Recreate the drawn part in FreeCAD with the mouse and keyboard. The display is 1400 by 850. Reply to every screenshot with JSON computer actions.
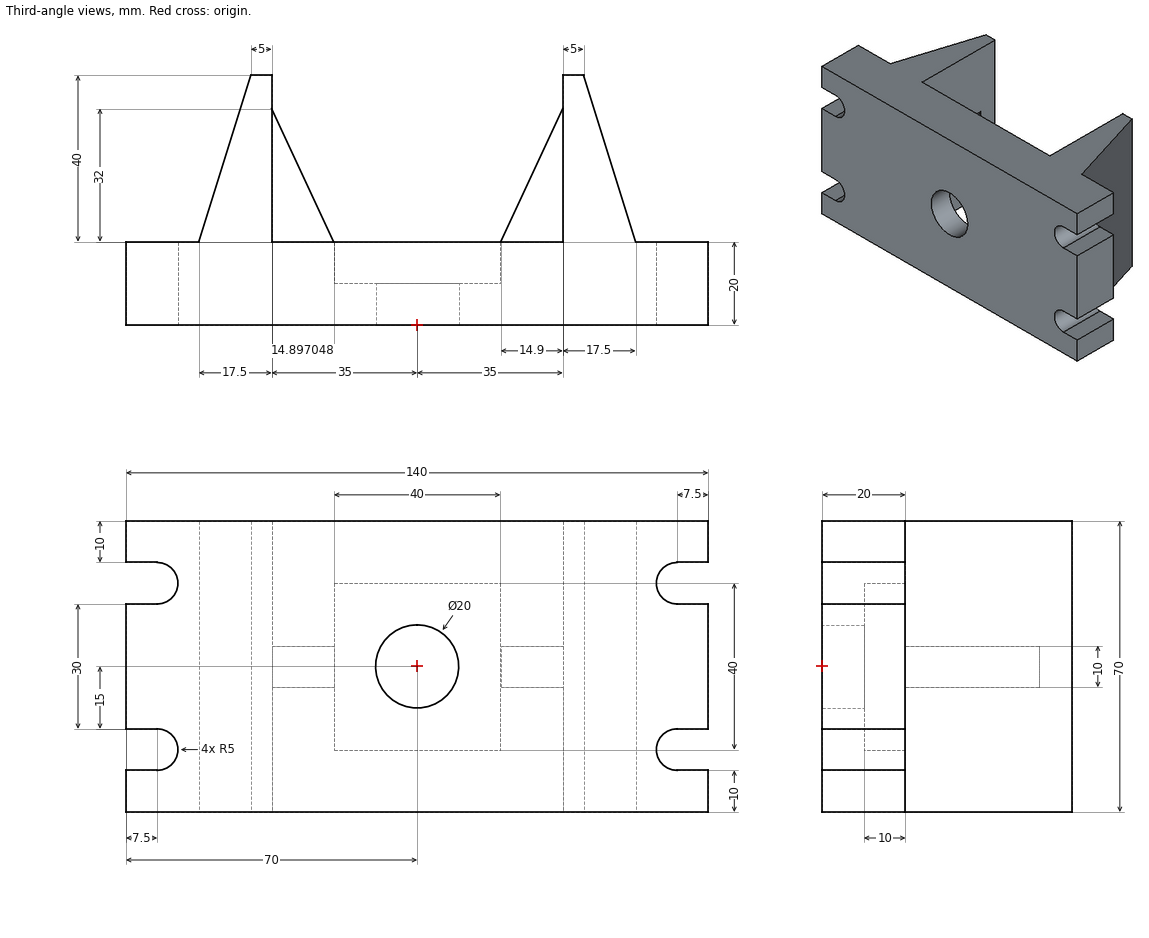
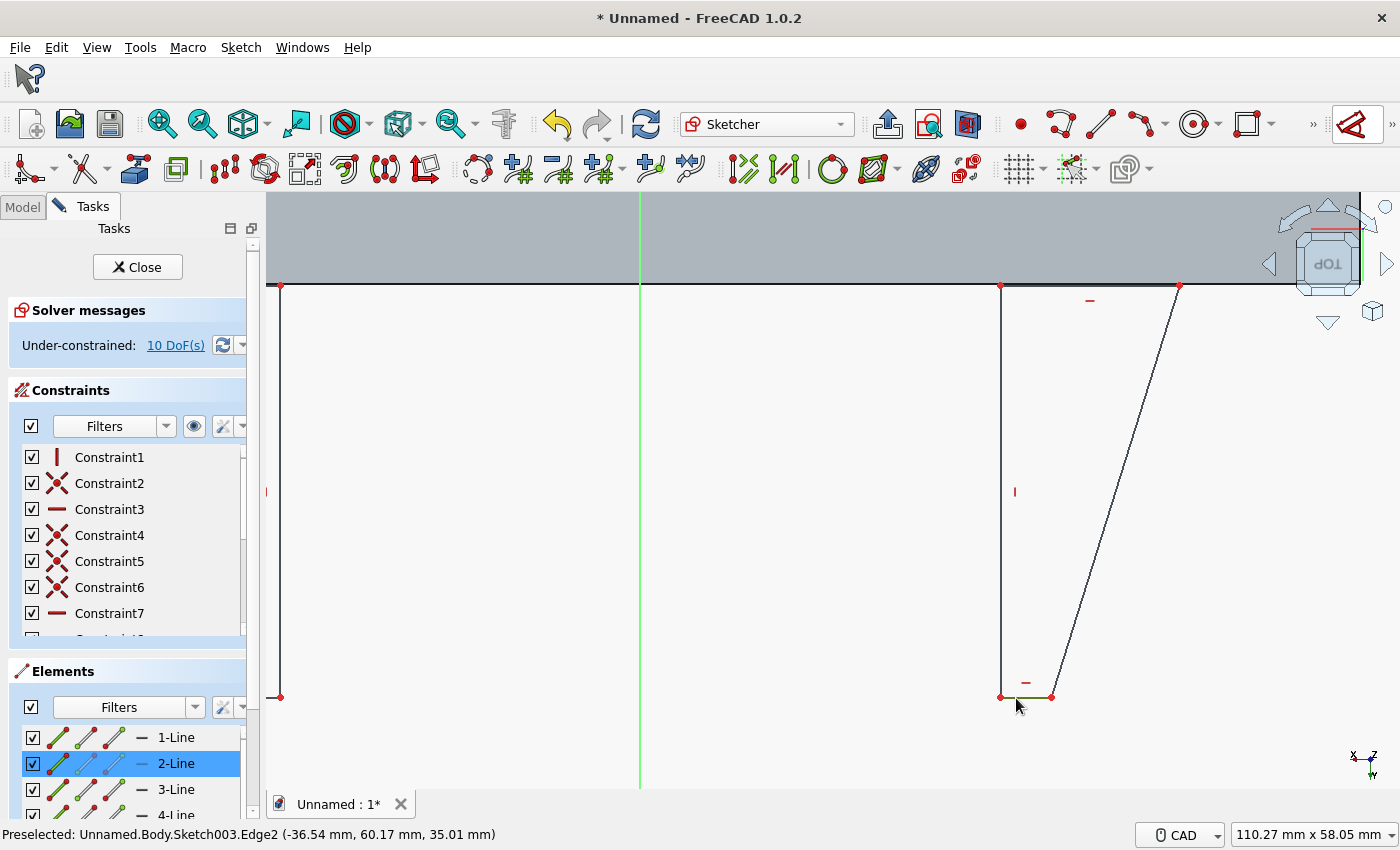
{"action": "left_click", "coordinate": [1378, 124]}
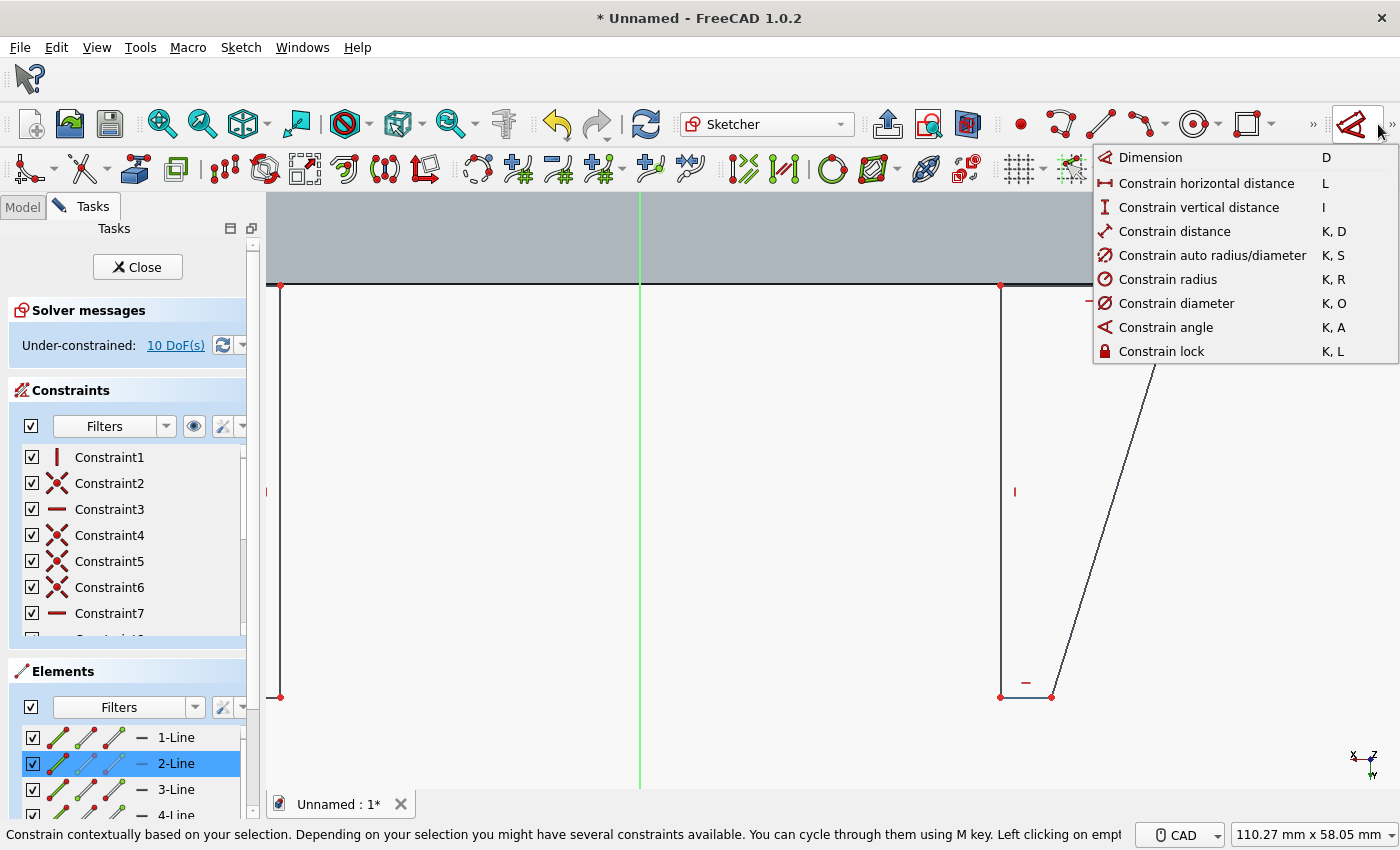
{"action": "left_click", "coordinate": [1246, 183]}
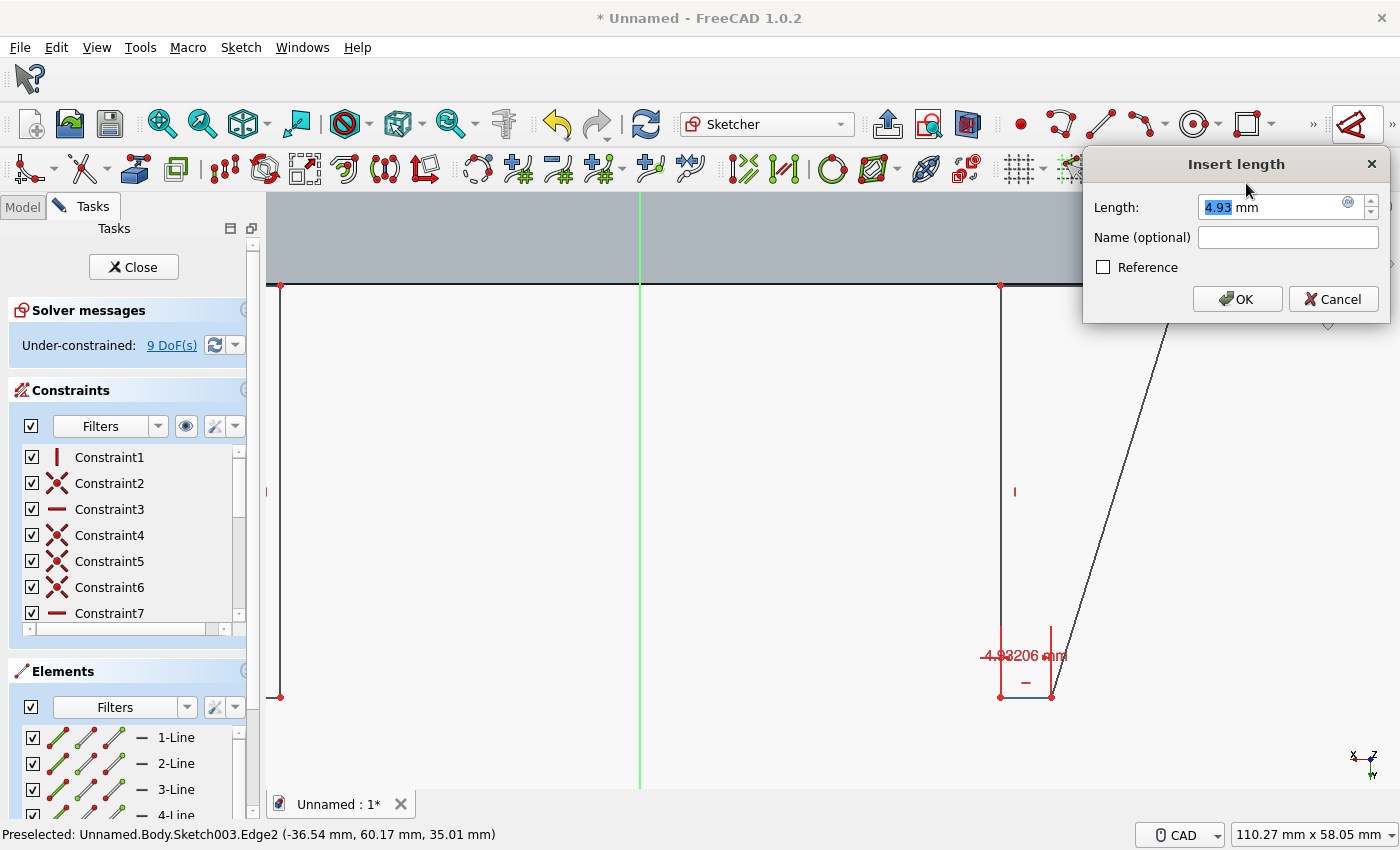
{"action": "type", "text": "5"}
{"action": "key", "text": "Return"}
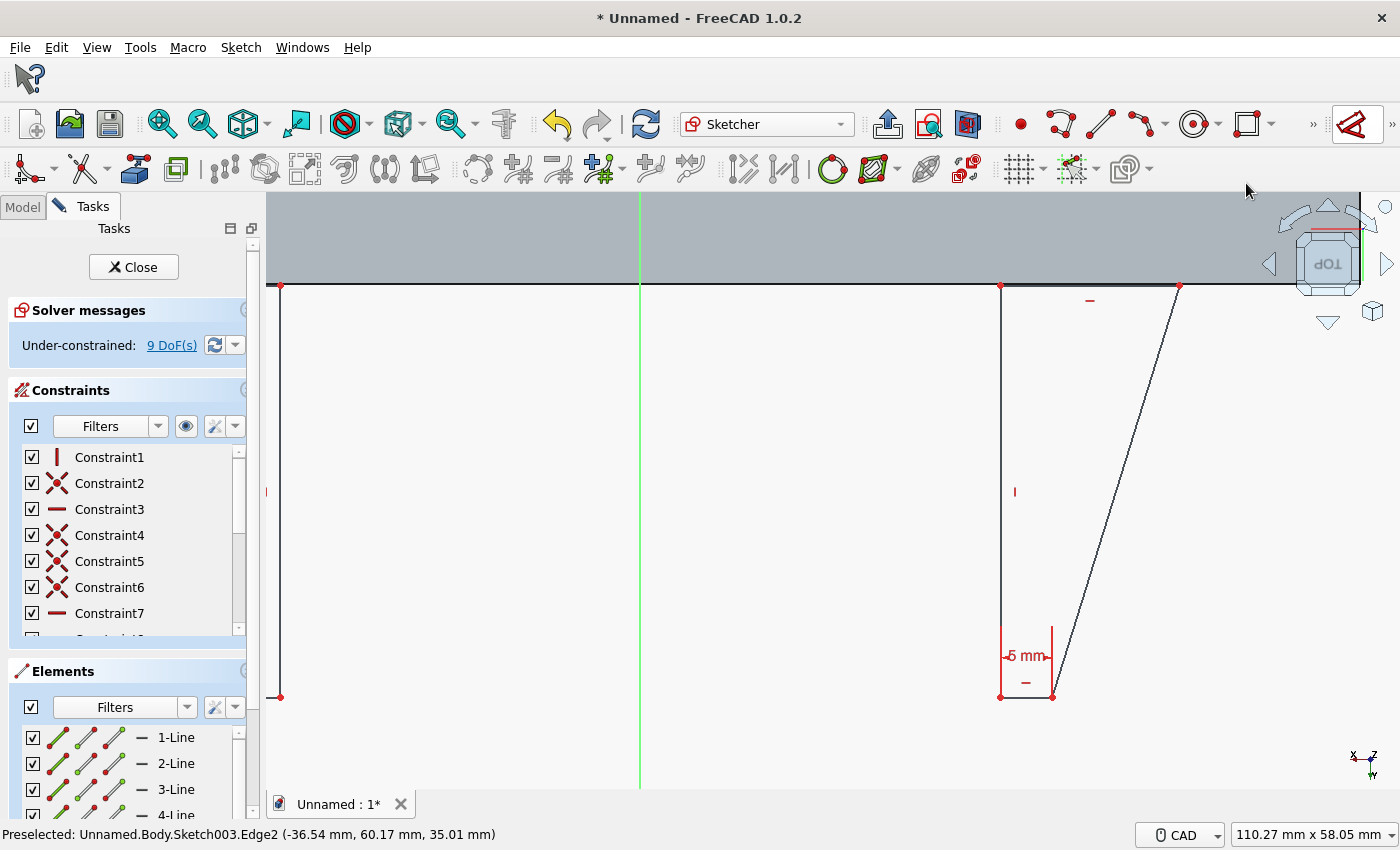
{"action": "scroll", "coordinate": [1017, 700], "scroll_direction": "down", "scroll_amount": 2}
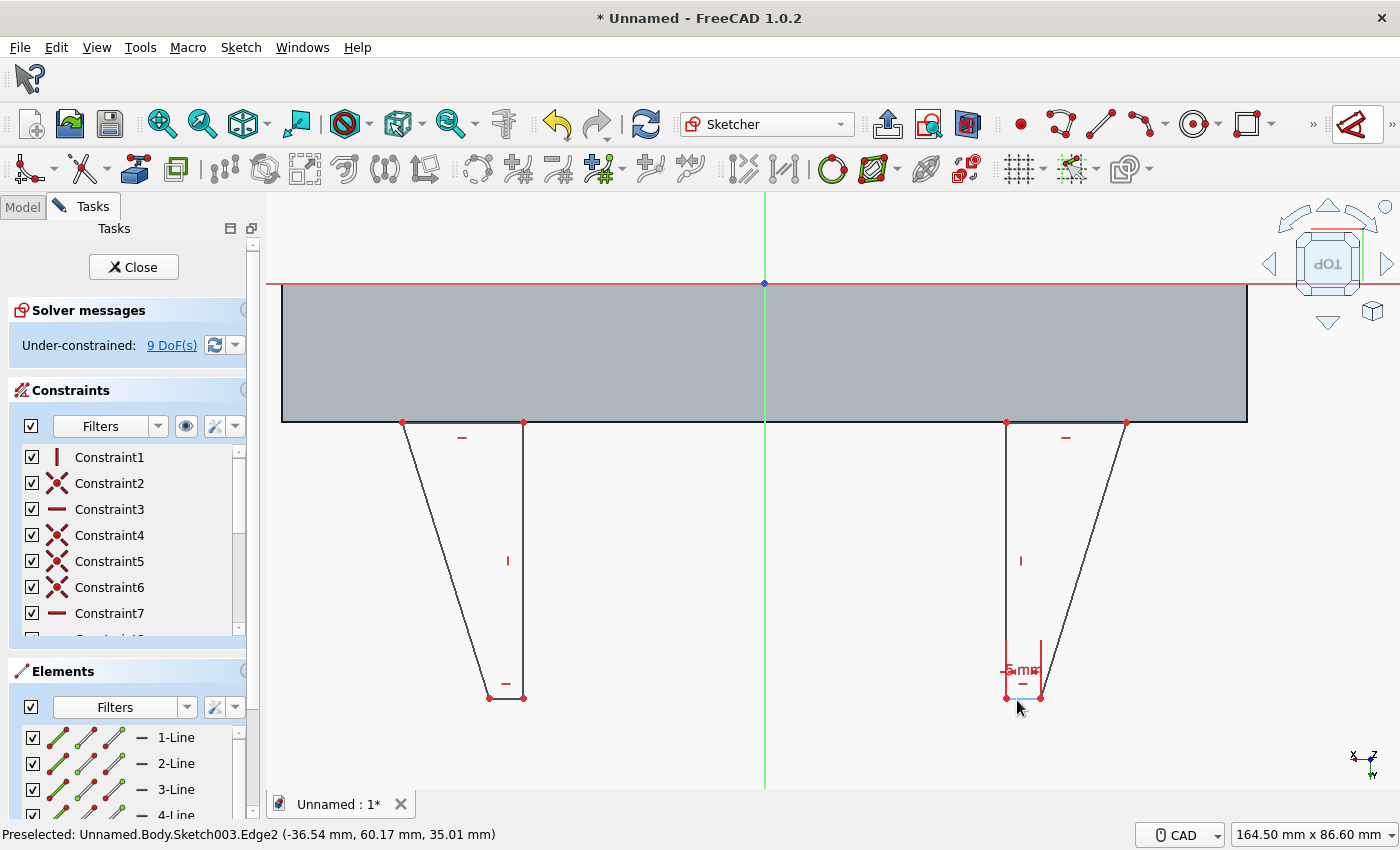
{"action": "scroll", "coordinate": [500, 699], "scroll_direction": "up", "scroll_amount": 2}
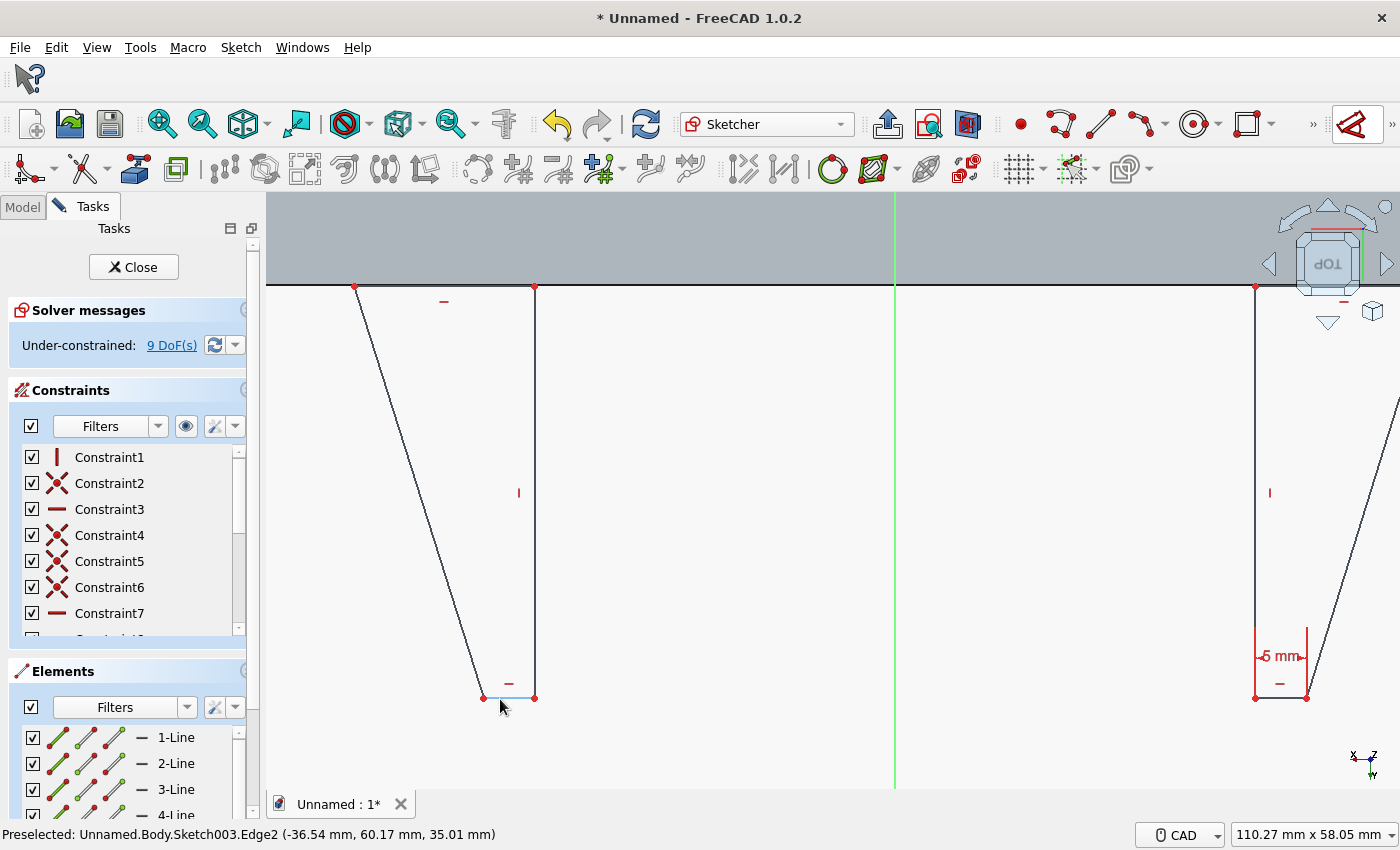
{"action": "left_click", "coordinate": [499, 698]}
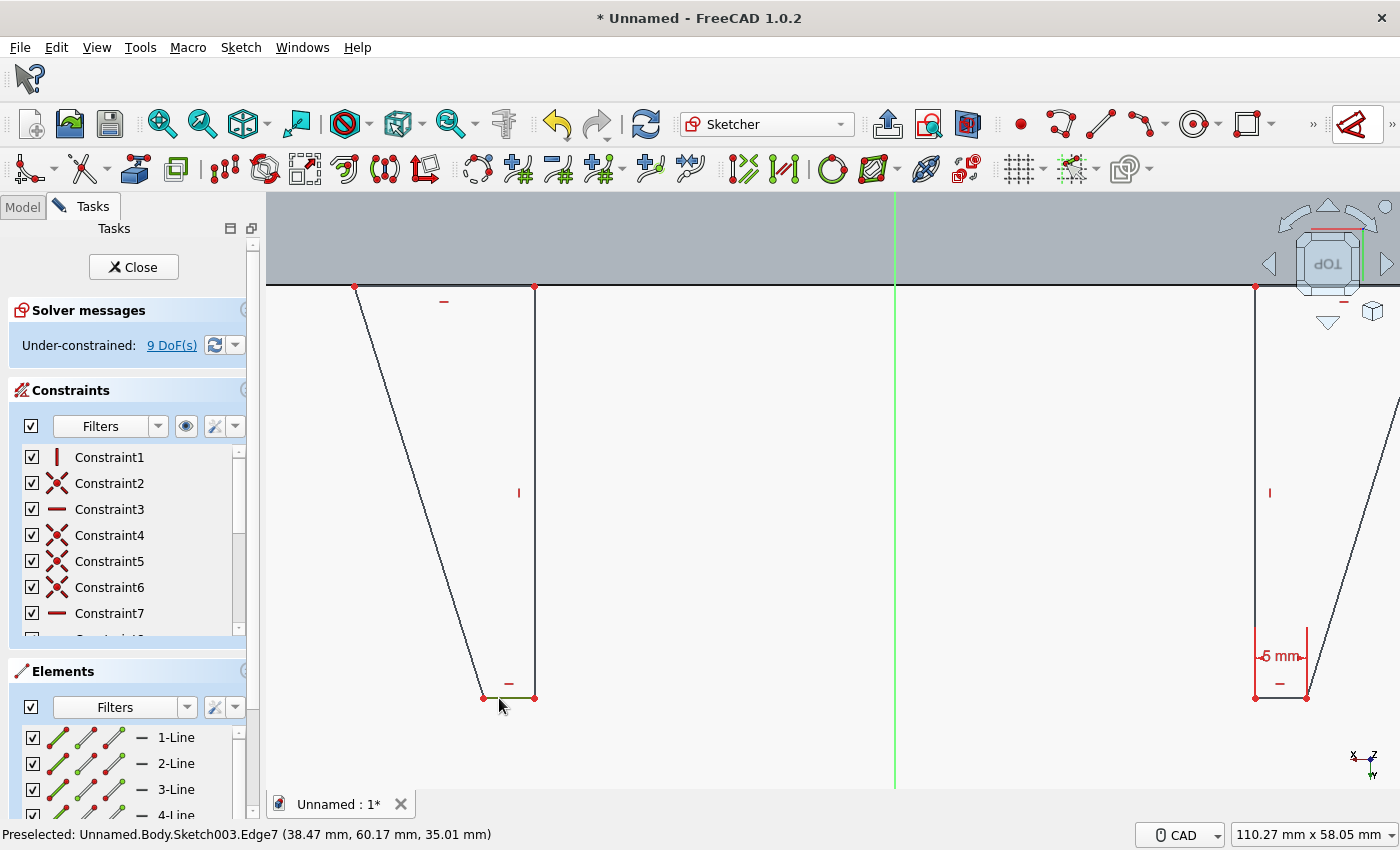
{"action": "key", "text": "l"}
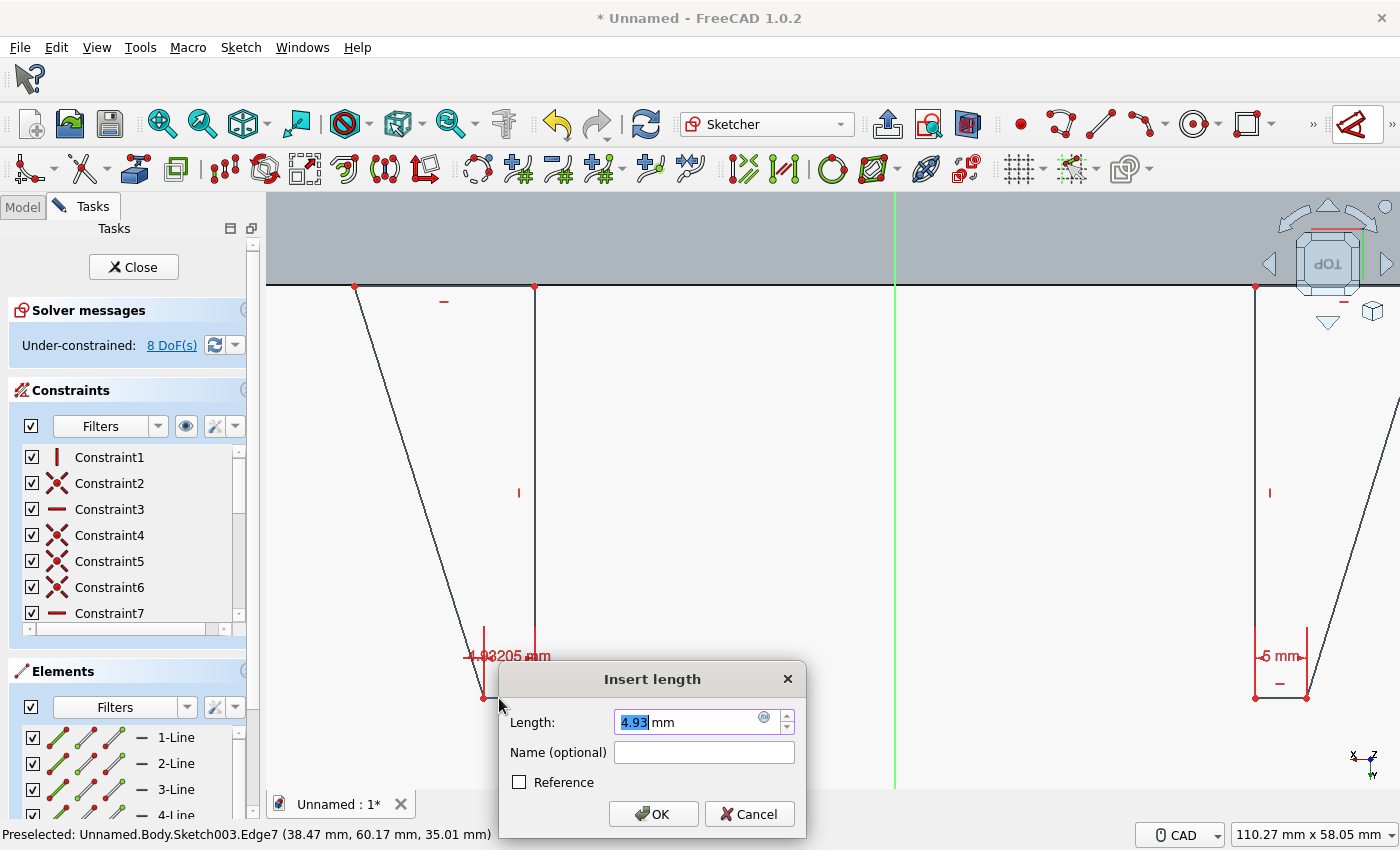
{"action": "type", "text": "5"}
{"action": "key", "text": "Return"}